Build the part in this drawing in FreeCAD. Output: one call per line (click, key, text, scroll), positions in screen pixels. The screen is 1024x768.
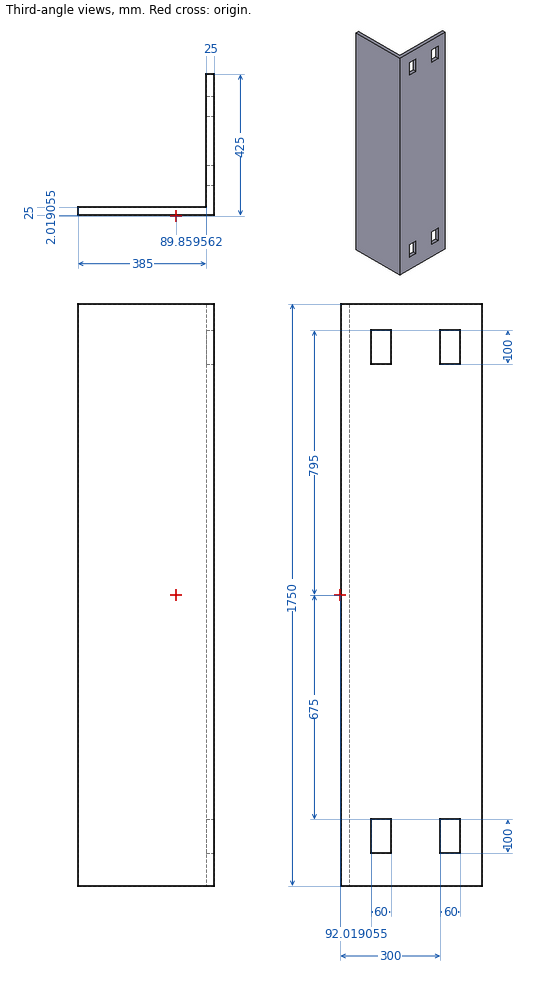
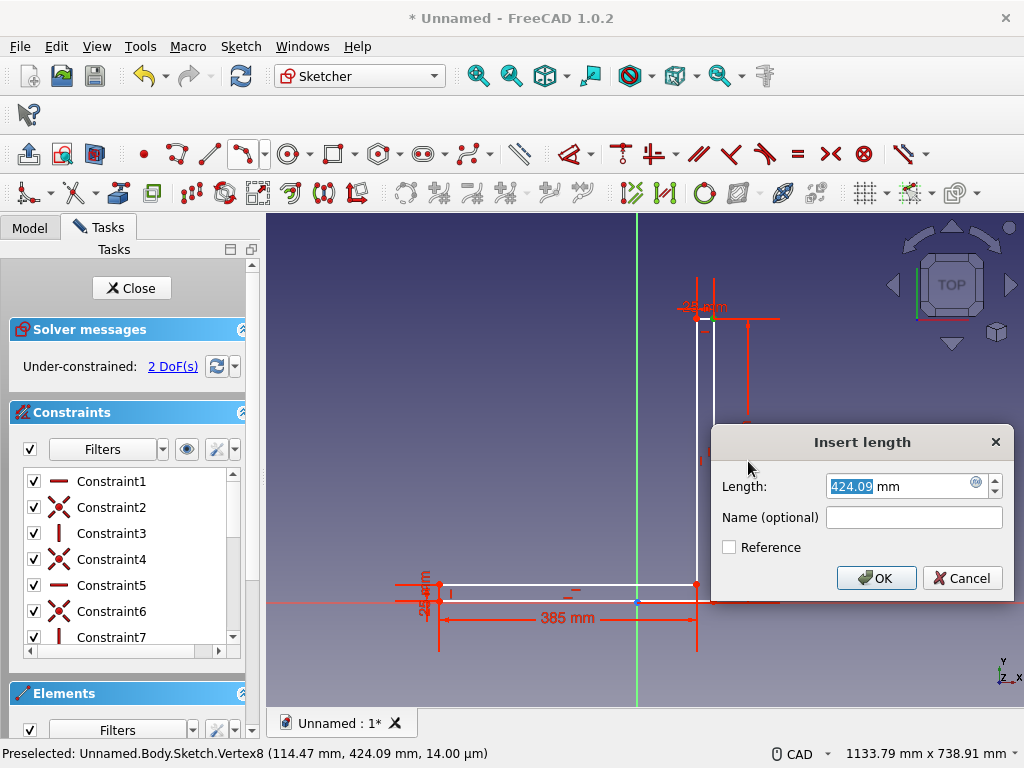
text(425)
key(Return)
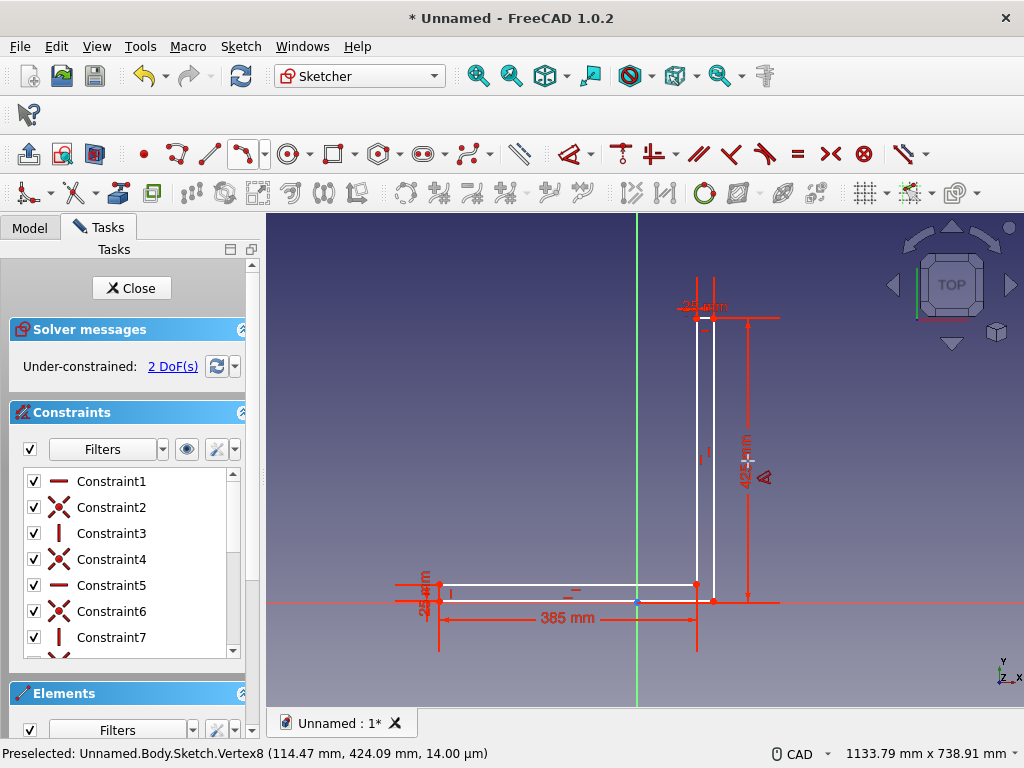
scroll(439, 601, up, 17)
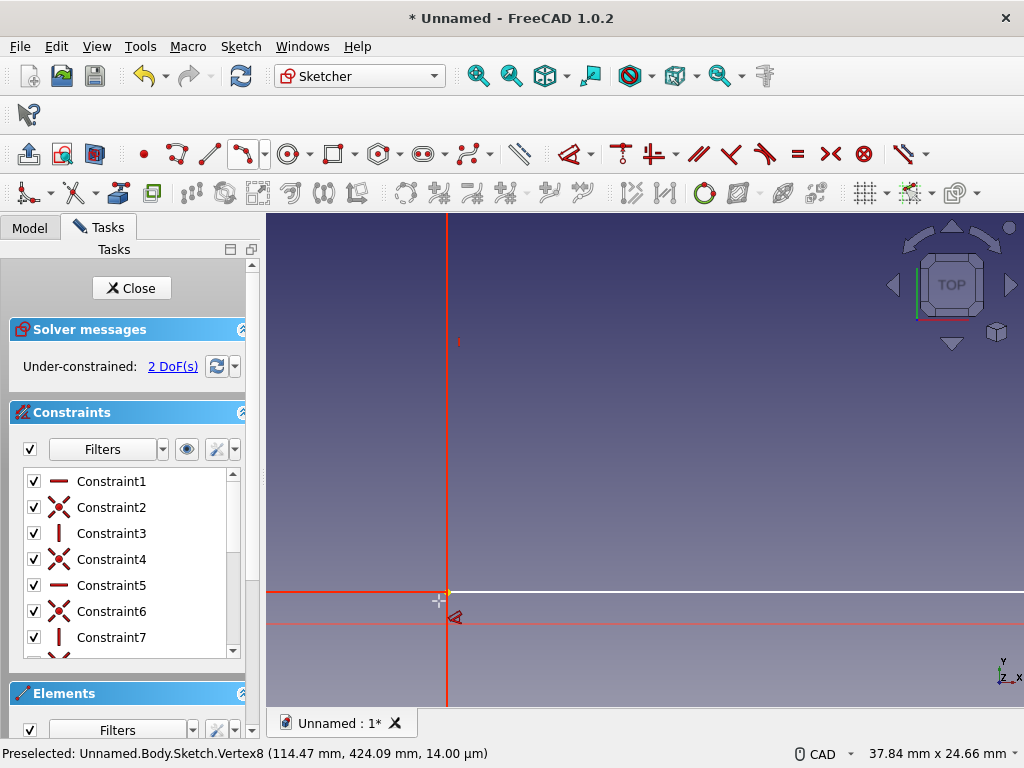
click(447, 592)
click(413, 608)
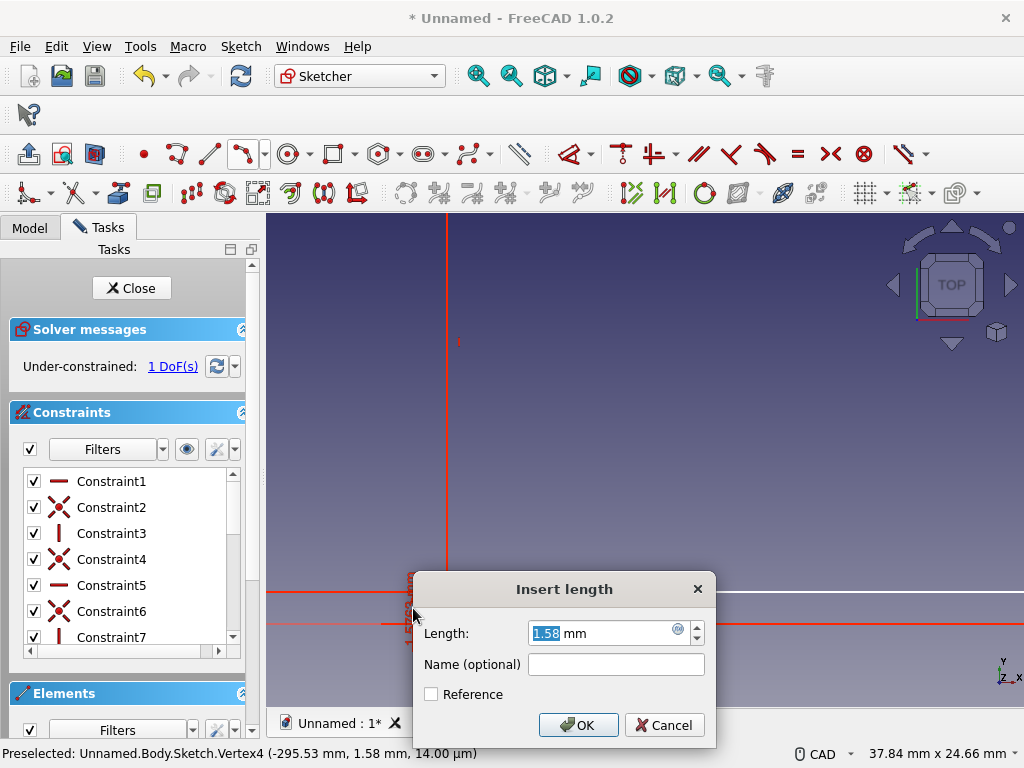
text(2.019055)
key(Return)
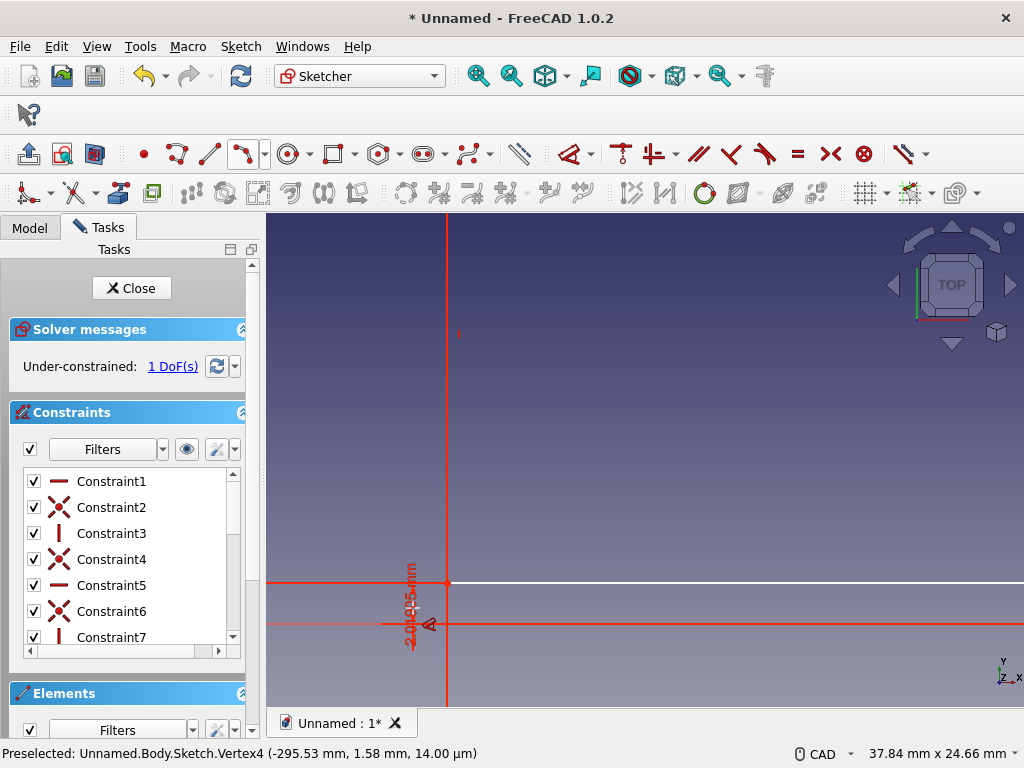
scroll(407, 634, down, 16)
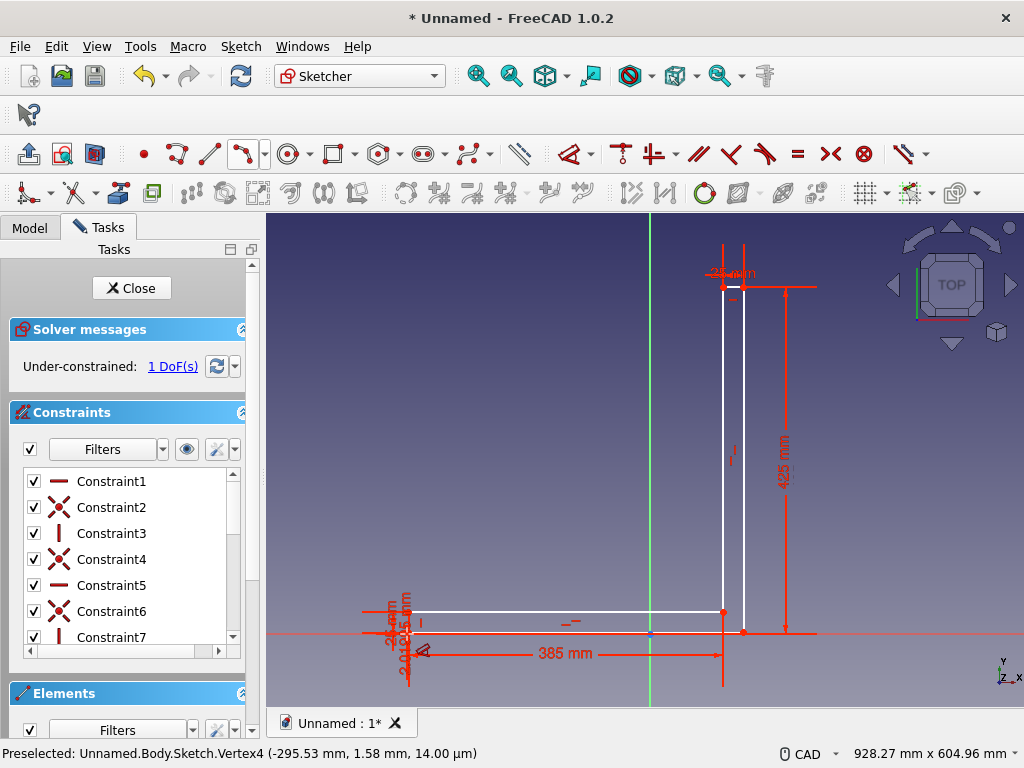
click(723, 612)
click(687, 668)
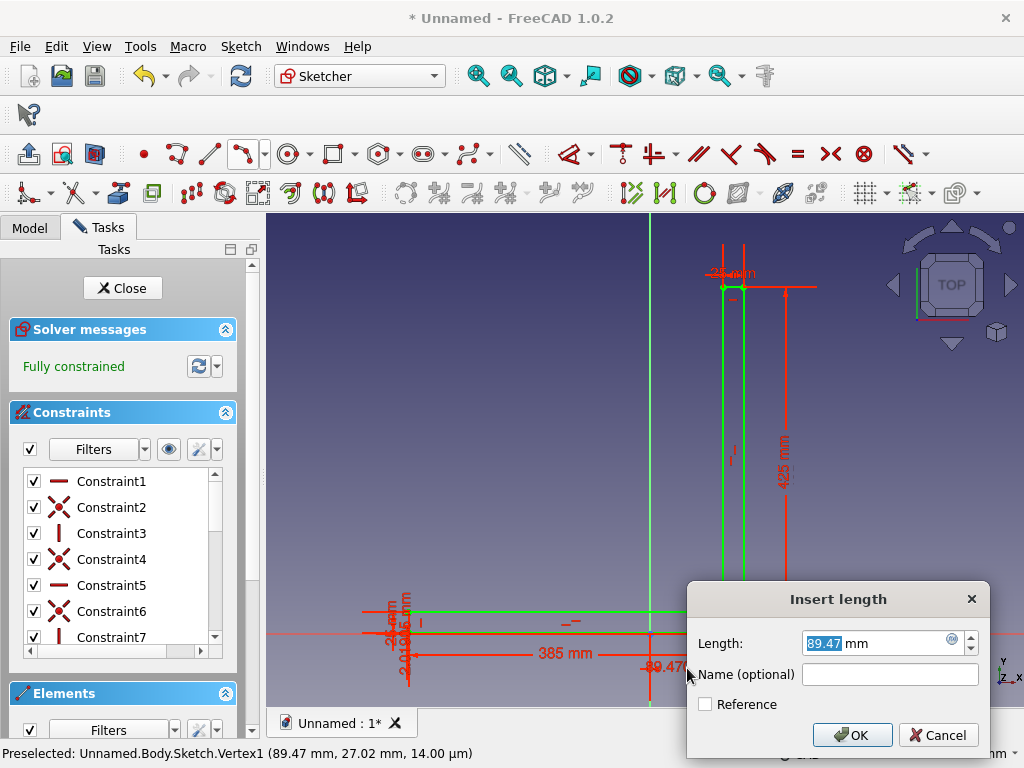
text(89.859562)
key(Return)
key(Escape)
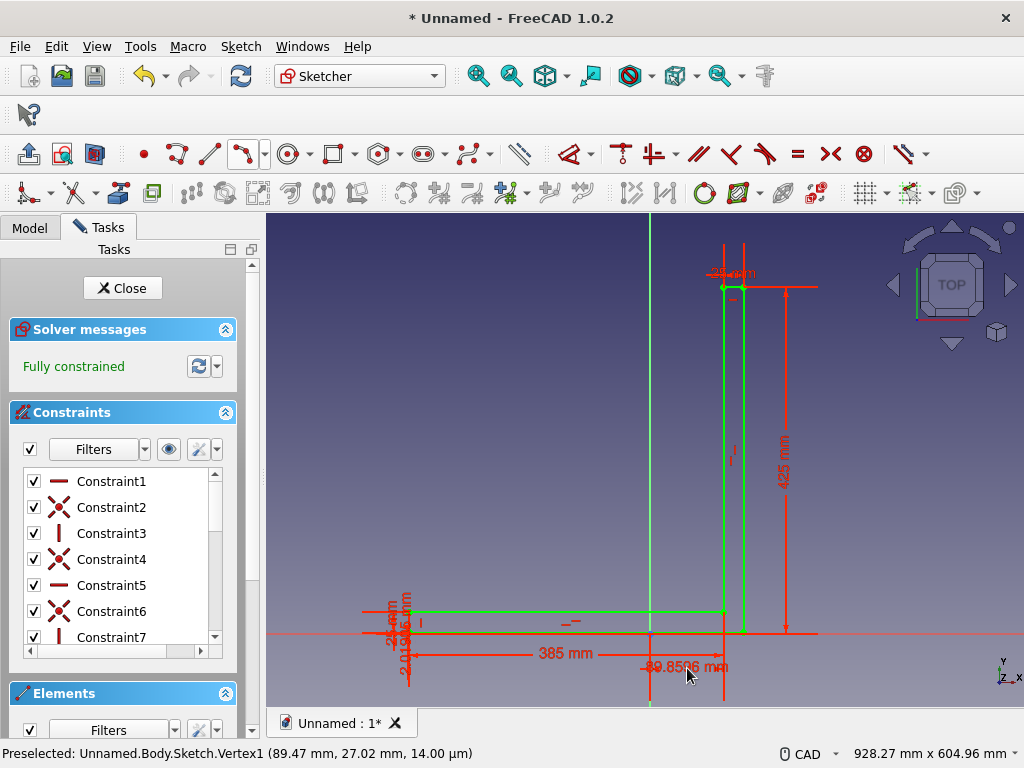
click(123, 288)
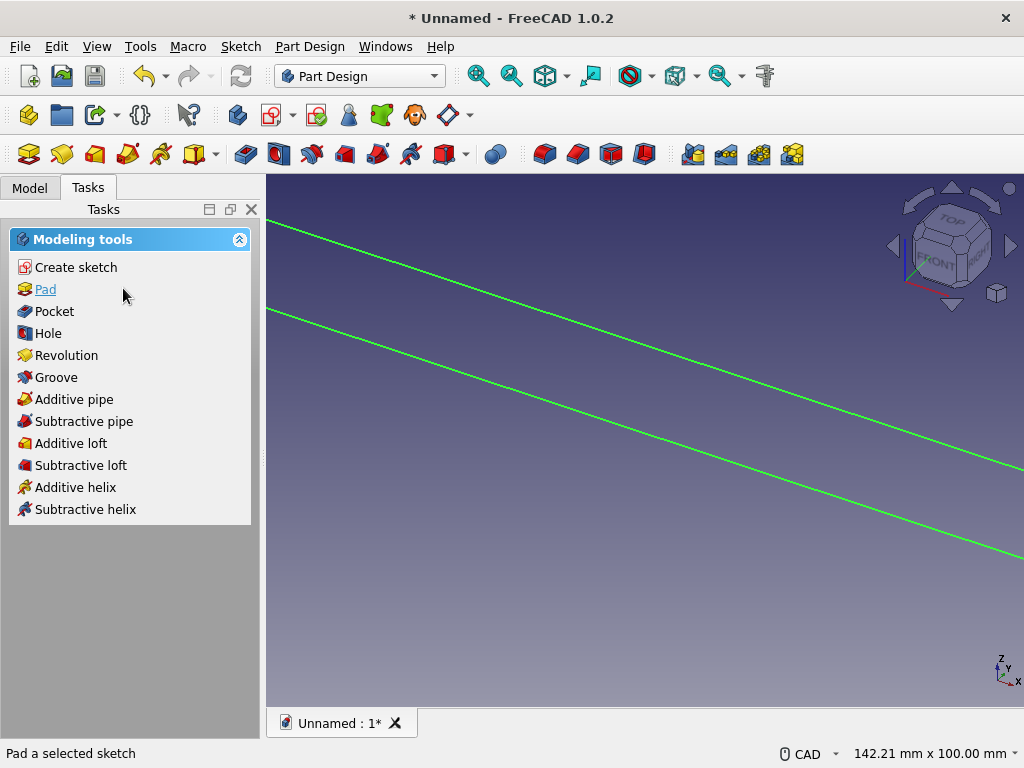
click(29, 154)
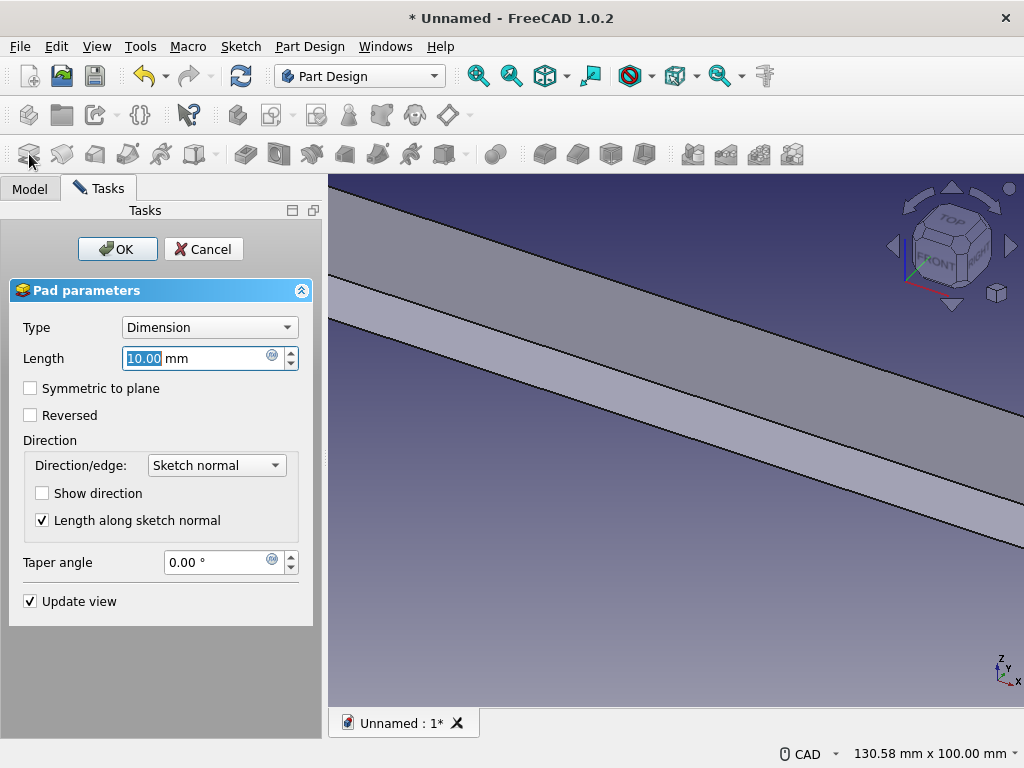
text(1750)
key(Tab)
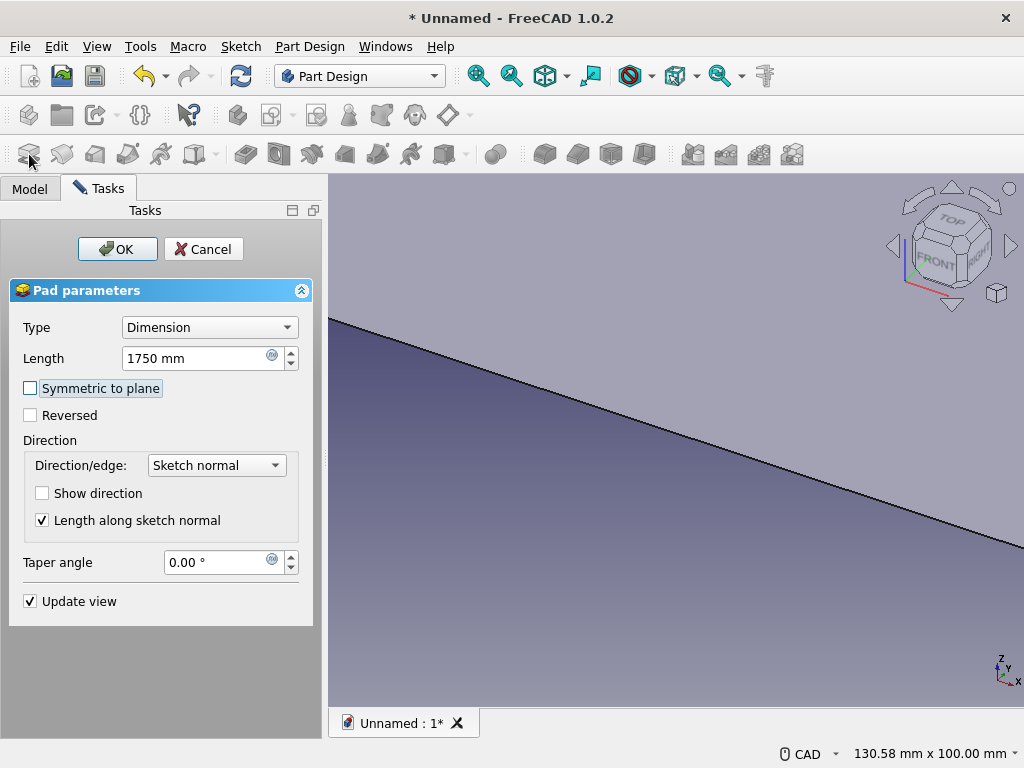
click(31, 388)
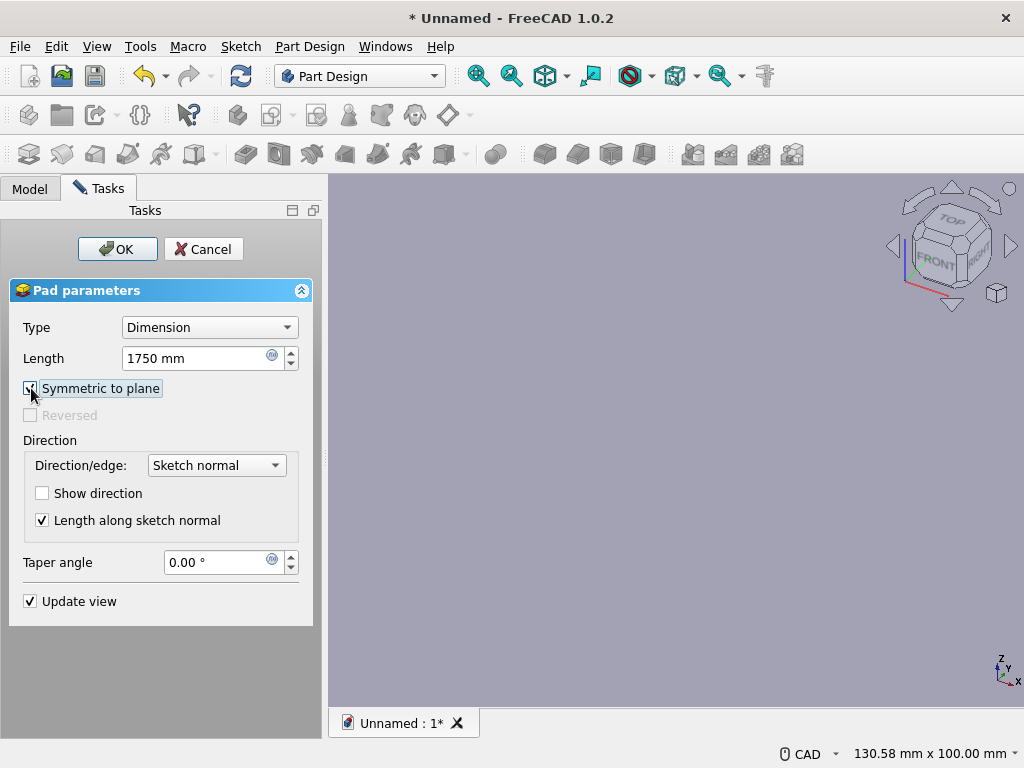
click(118, 249)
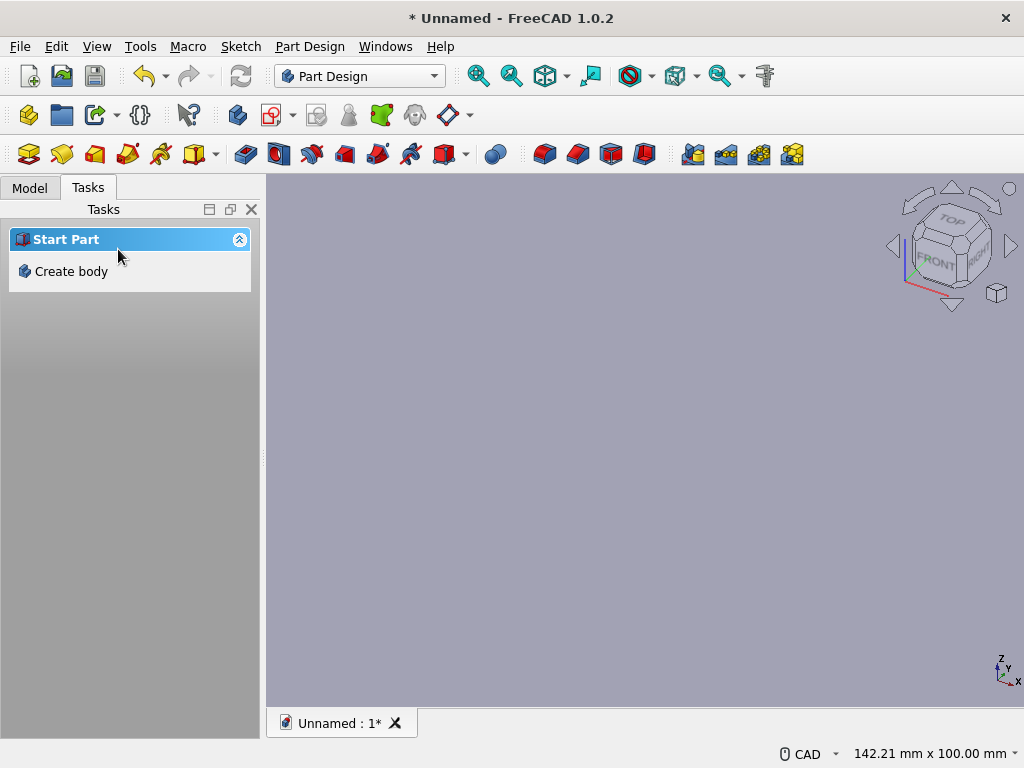
click(479, 76)